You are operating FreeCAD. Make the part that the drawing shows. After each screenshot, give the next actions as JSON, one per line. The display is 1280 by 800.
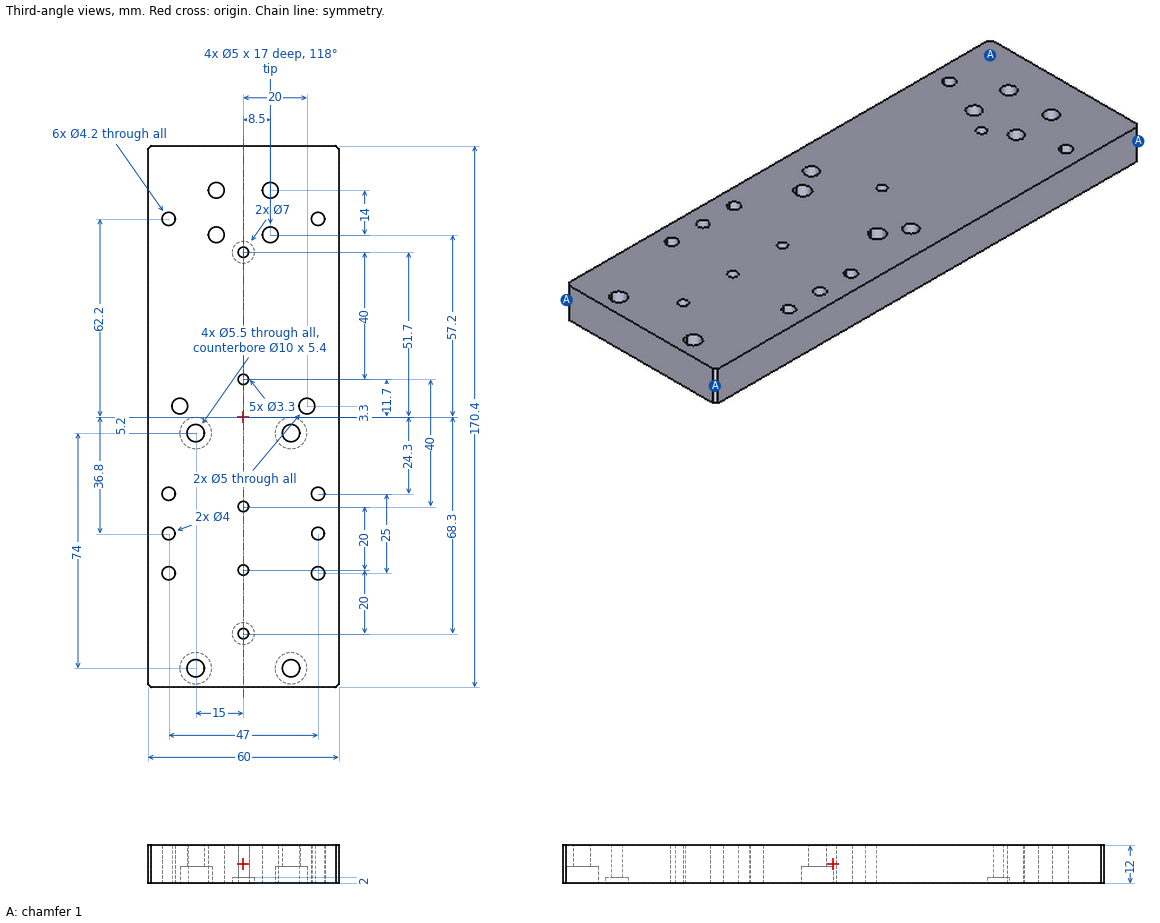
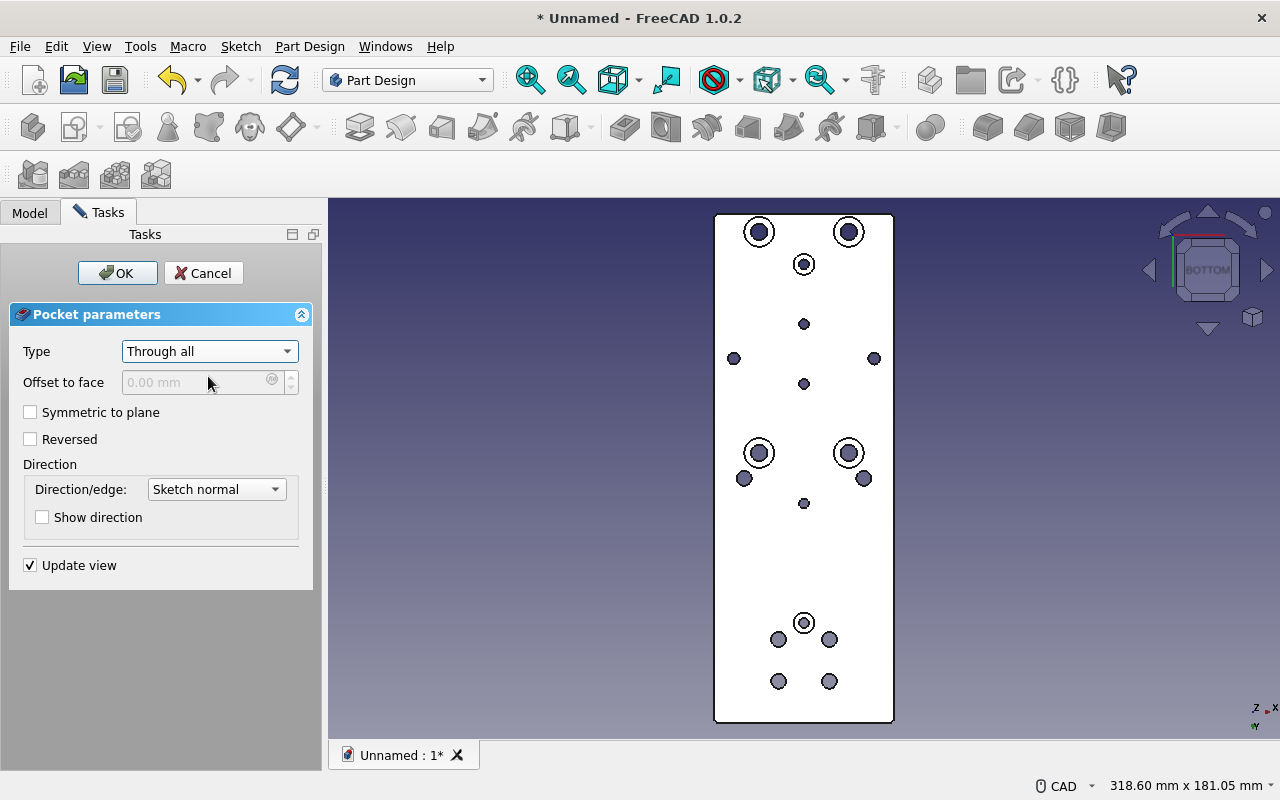
{"action": "left_click", "coordinate": [118, 273]}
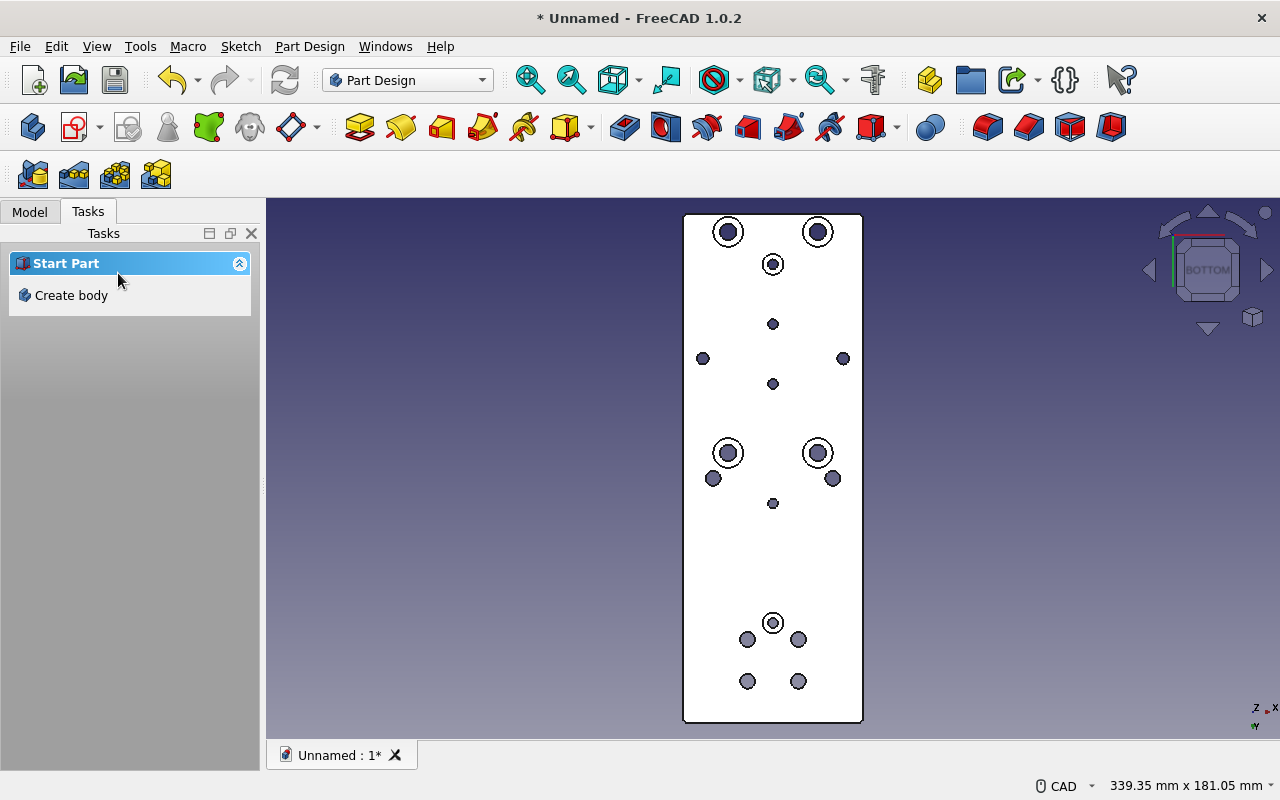
{"action": "left_click", "coordinate": [747, 540]}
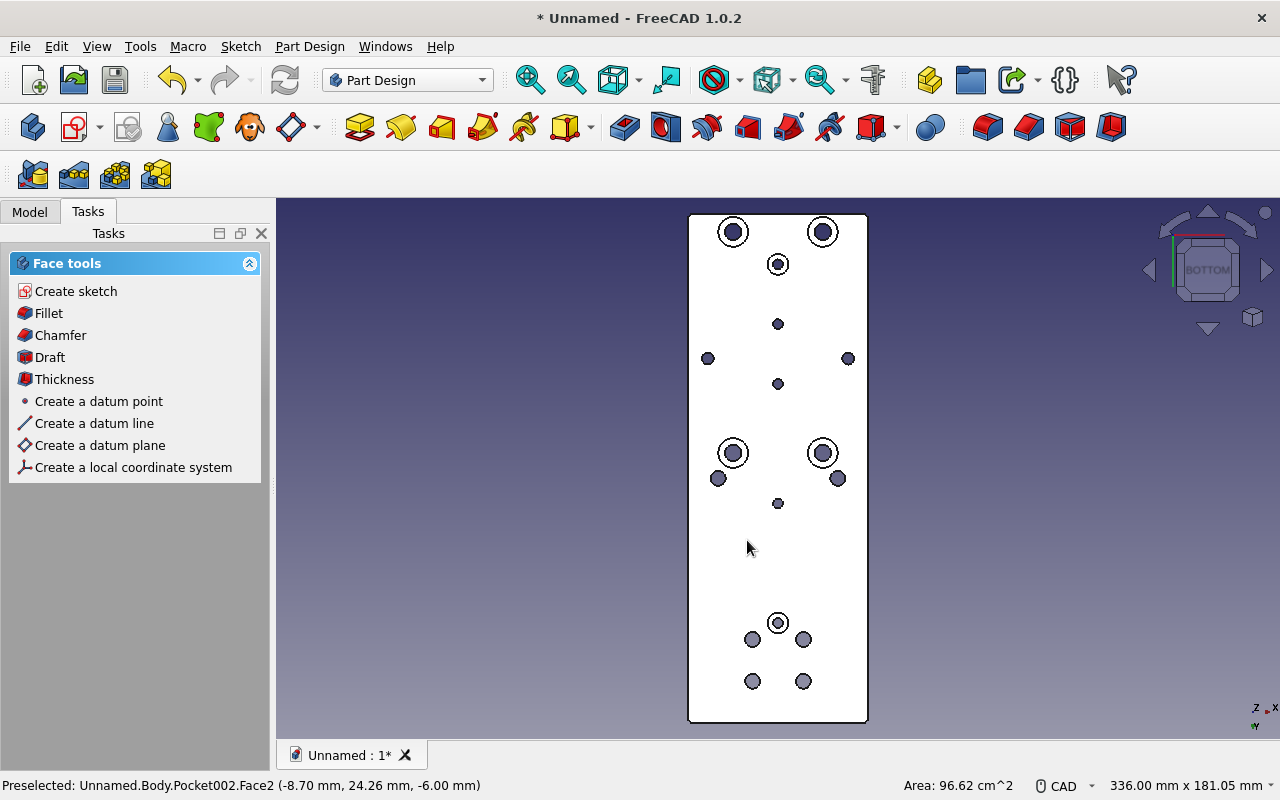
{"action": "left_click", "coordinate": [74, 128]}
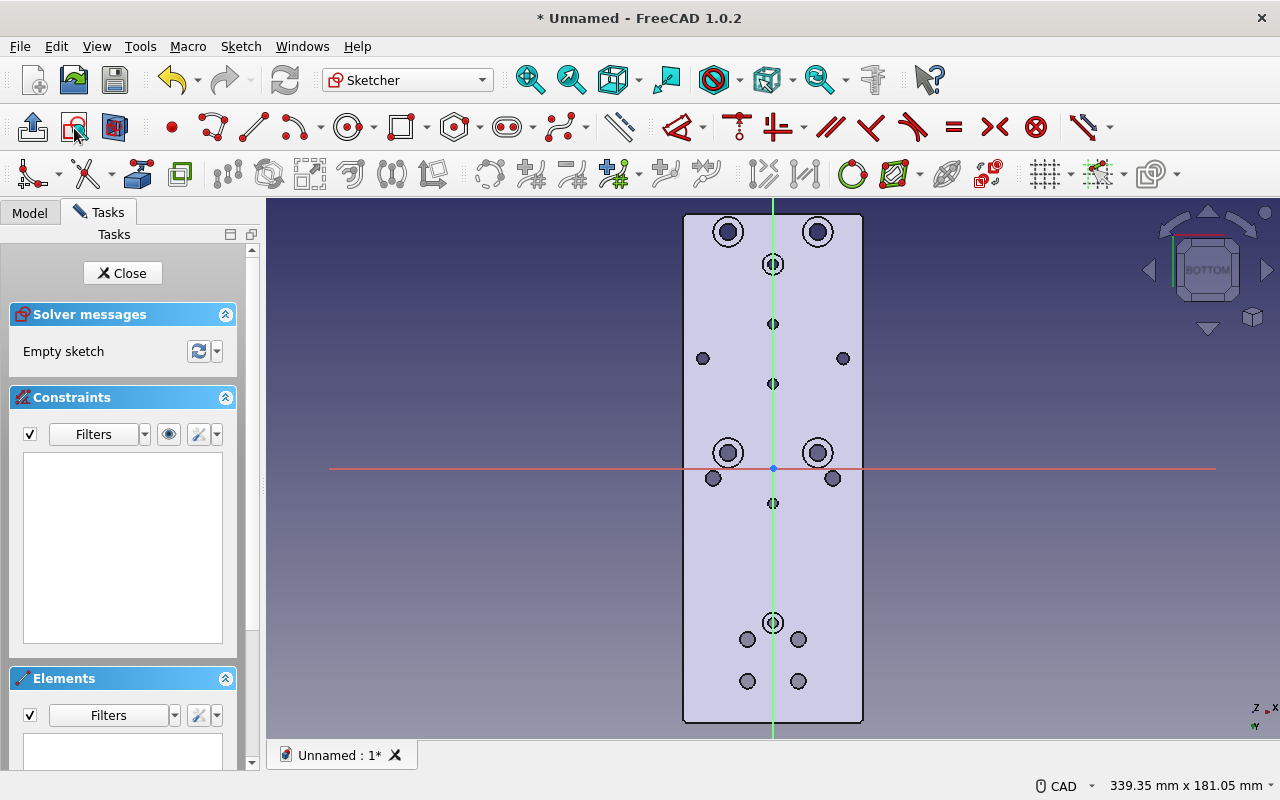
{"action": "left_click", "coordinate": [348, 128]}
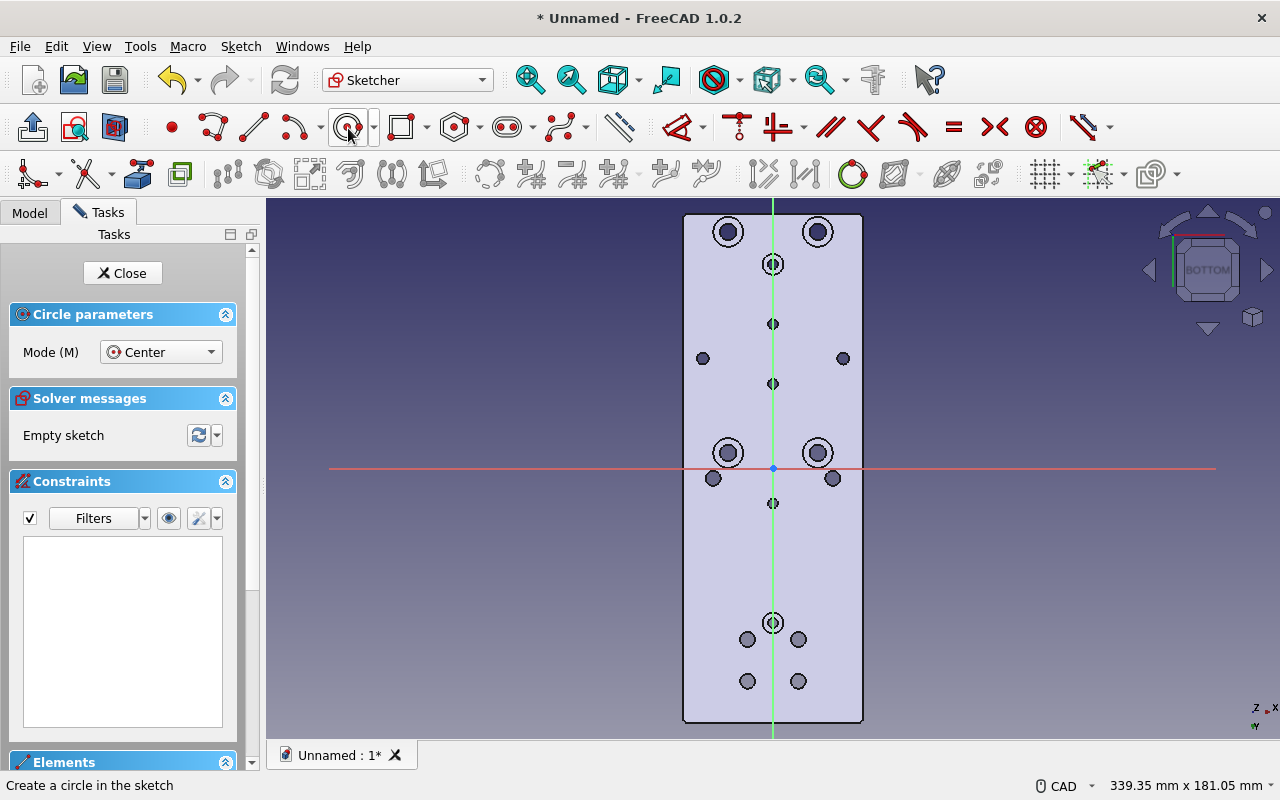
{"action": "scroll", "coordinate": [703, 654], "scroll_direction": "up", "scroll_amount": 7}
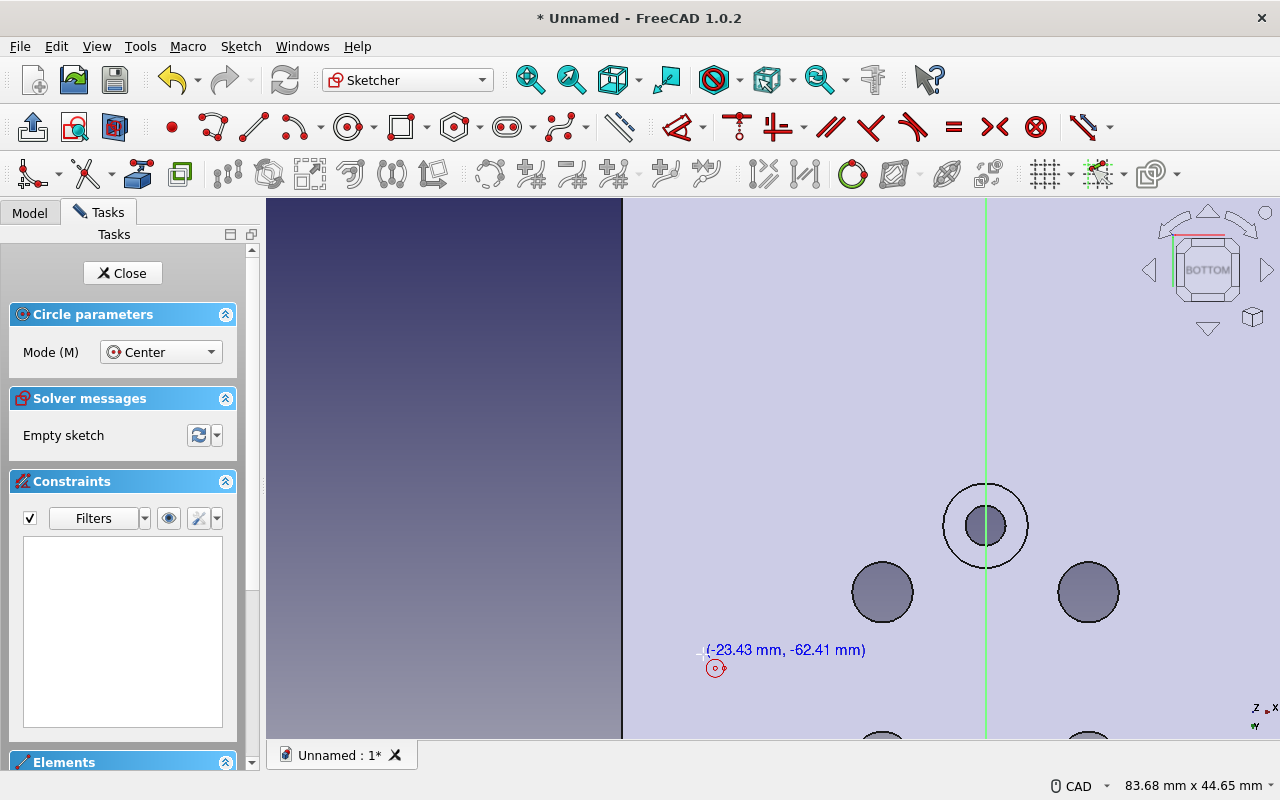
{"action": "scroll", "coordinate": [613, 629], "scroll_direction": "down", "scroll_amount": 7}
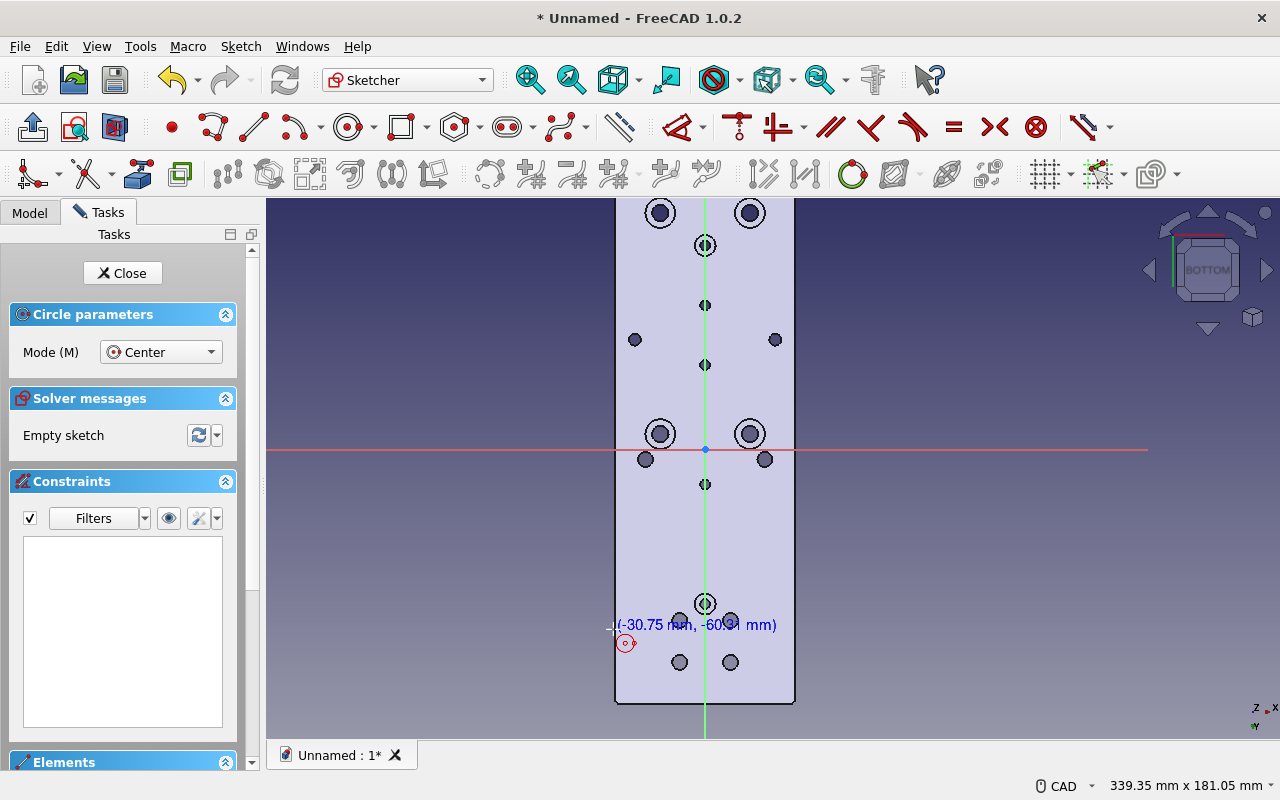
{"action": "left_click", "coordinate": [635, 635]}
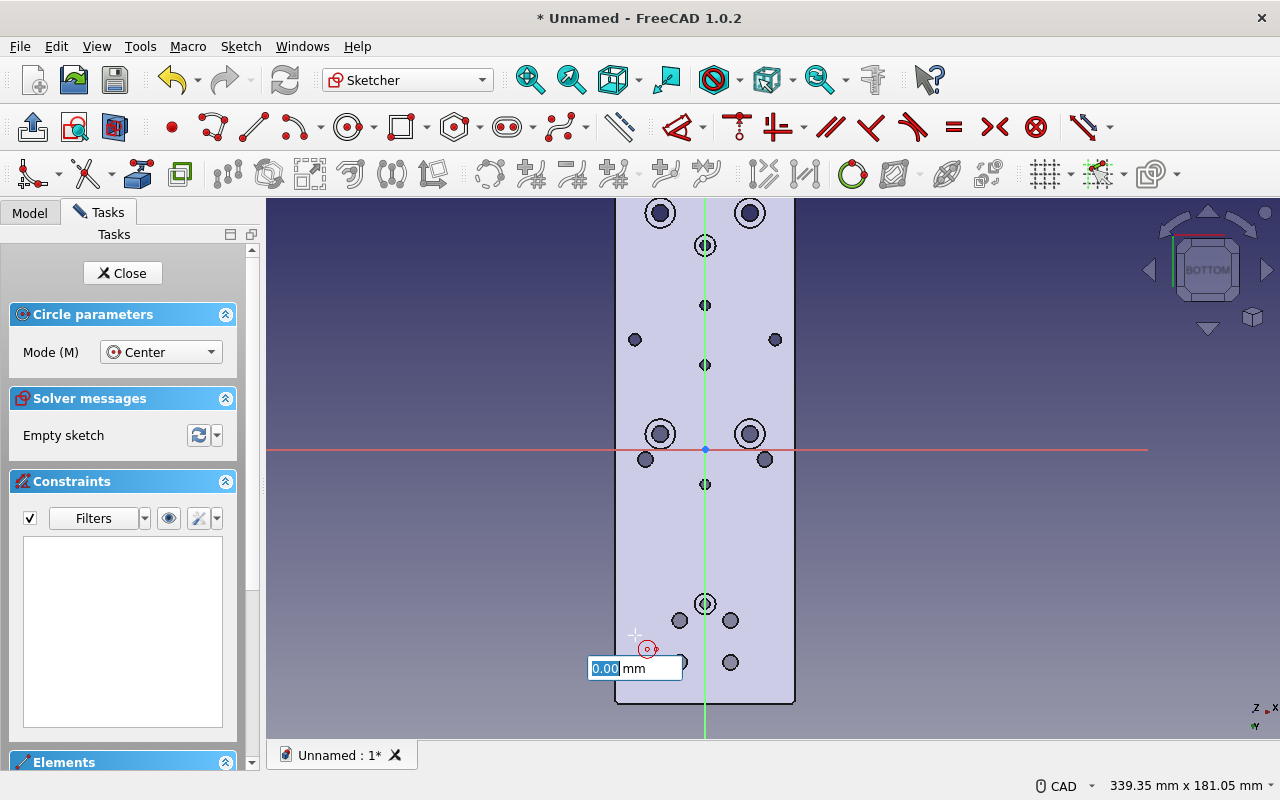
{"action": "scroll", "coordinate": [639, 631], "scroll_direction": "up", "scroll_amount": 5}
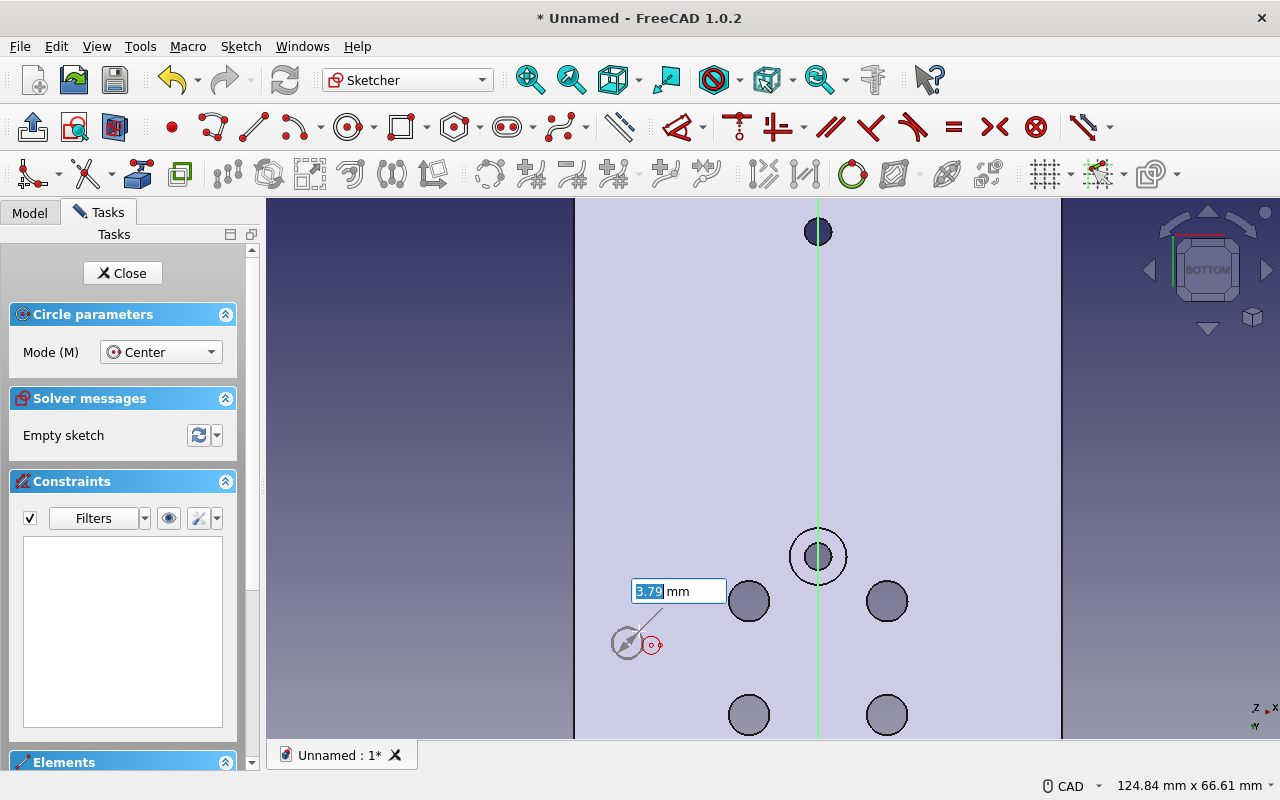
{"action": "left_click", "coordinate": [639, 630]}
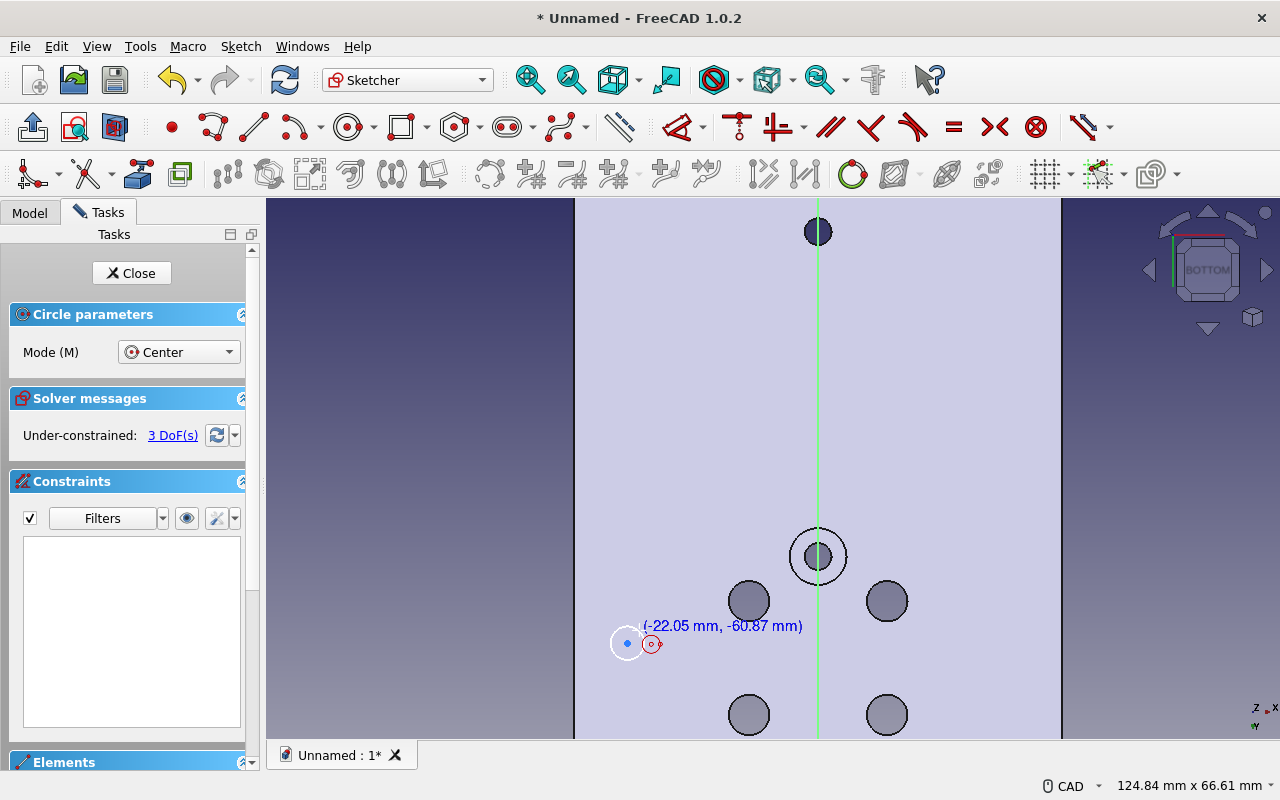
{"action": "scroll", "coordinate": [638, 631], "scroll_direction": "down", "scroll_amount": 5}